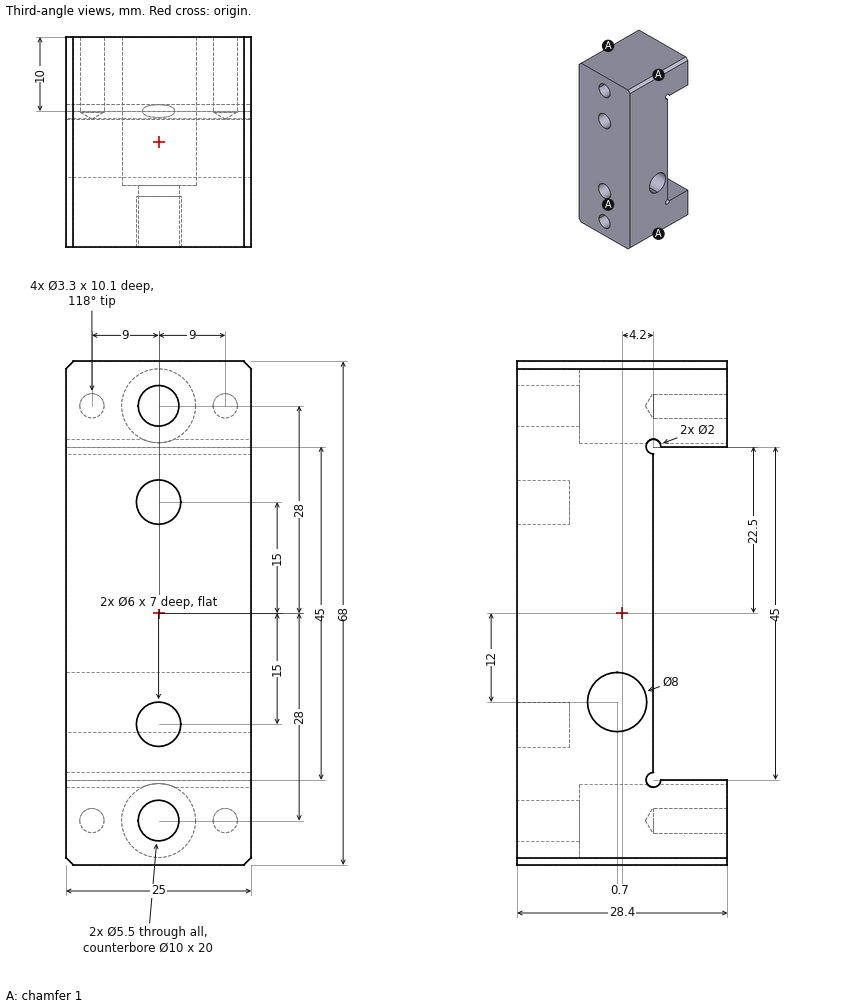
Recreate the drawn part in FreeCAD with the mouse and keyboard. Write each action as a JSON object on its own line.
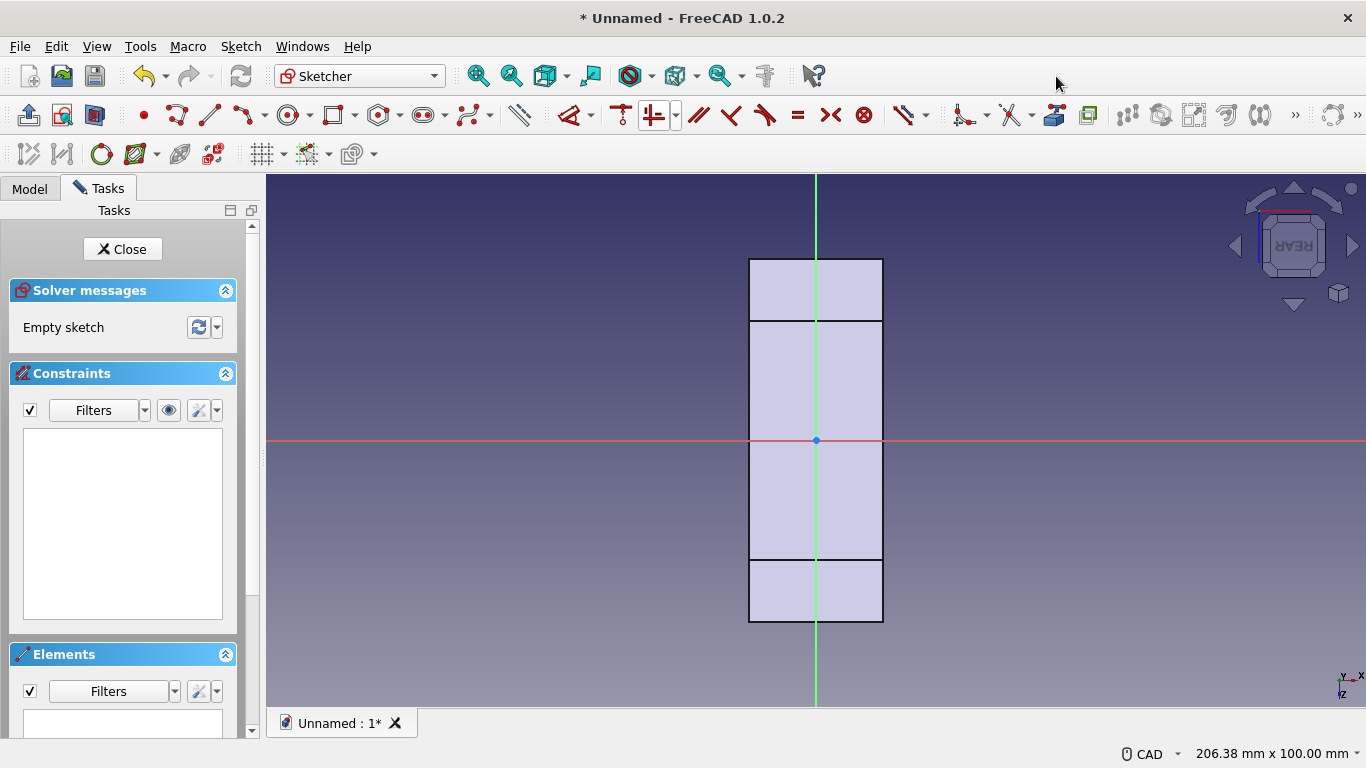
{"action": "key", "text": "g c"}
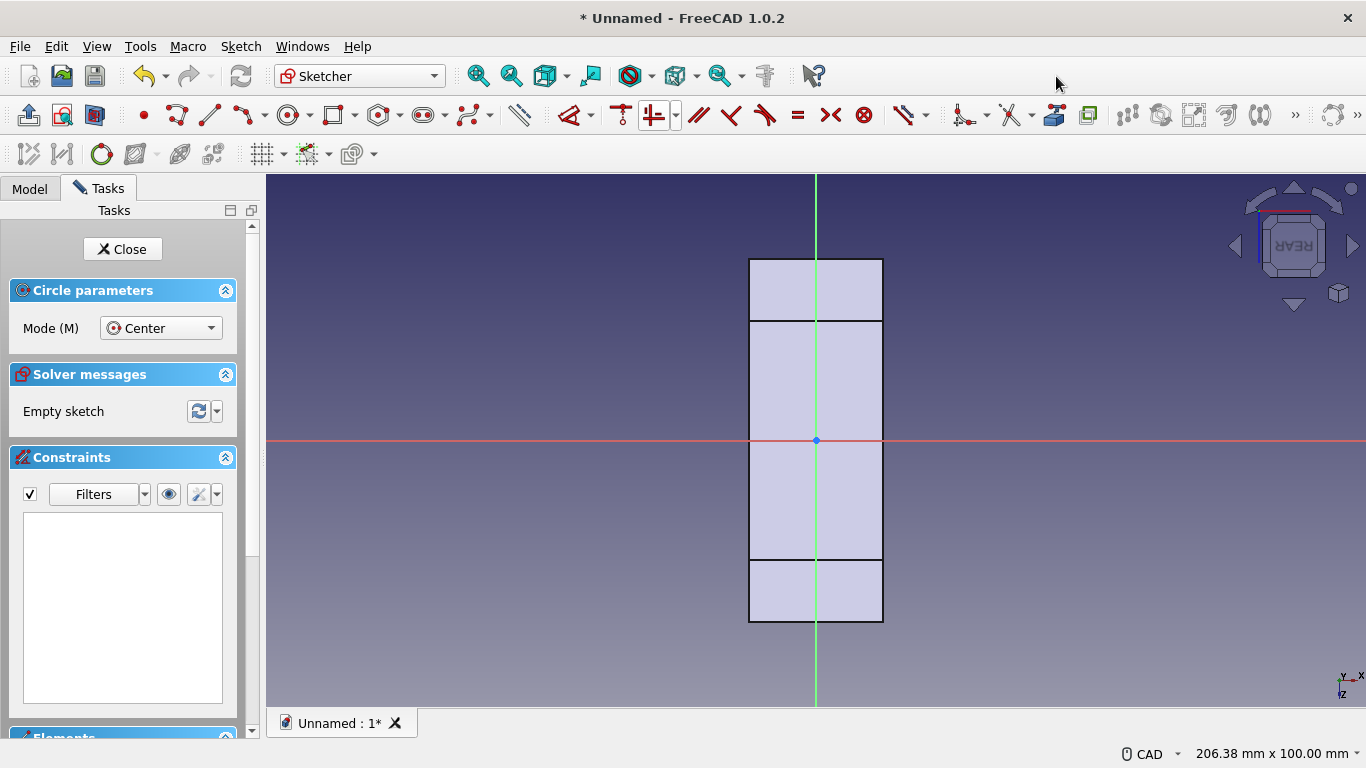
{"action": "scroll", "coordinate": [816, 291], "scroll_direction": "up", "scroll_amount": 3}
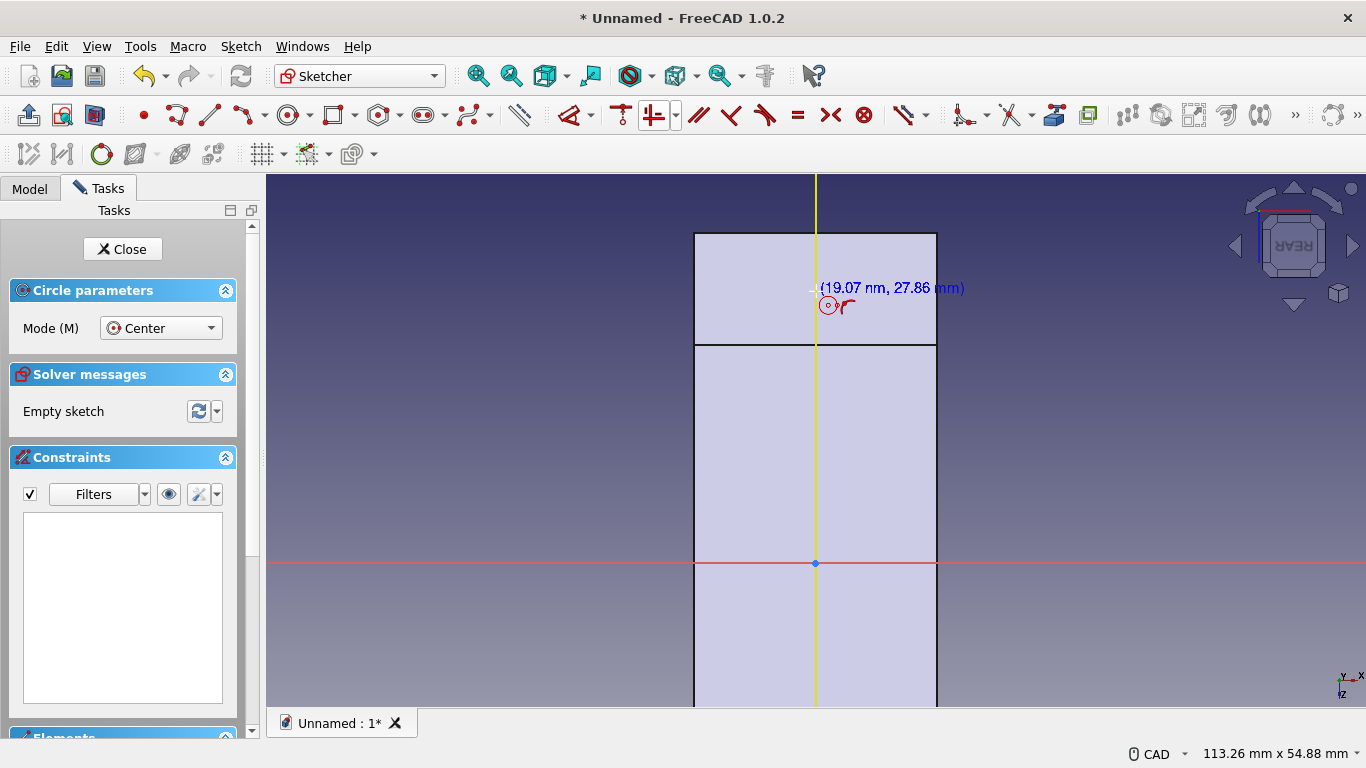
{"action": "left_click", "coordinate": [816, 291]}
{"action": "left_click", "coordinate": [834, 272]}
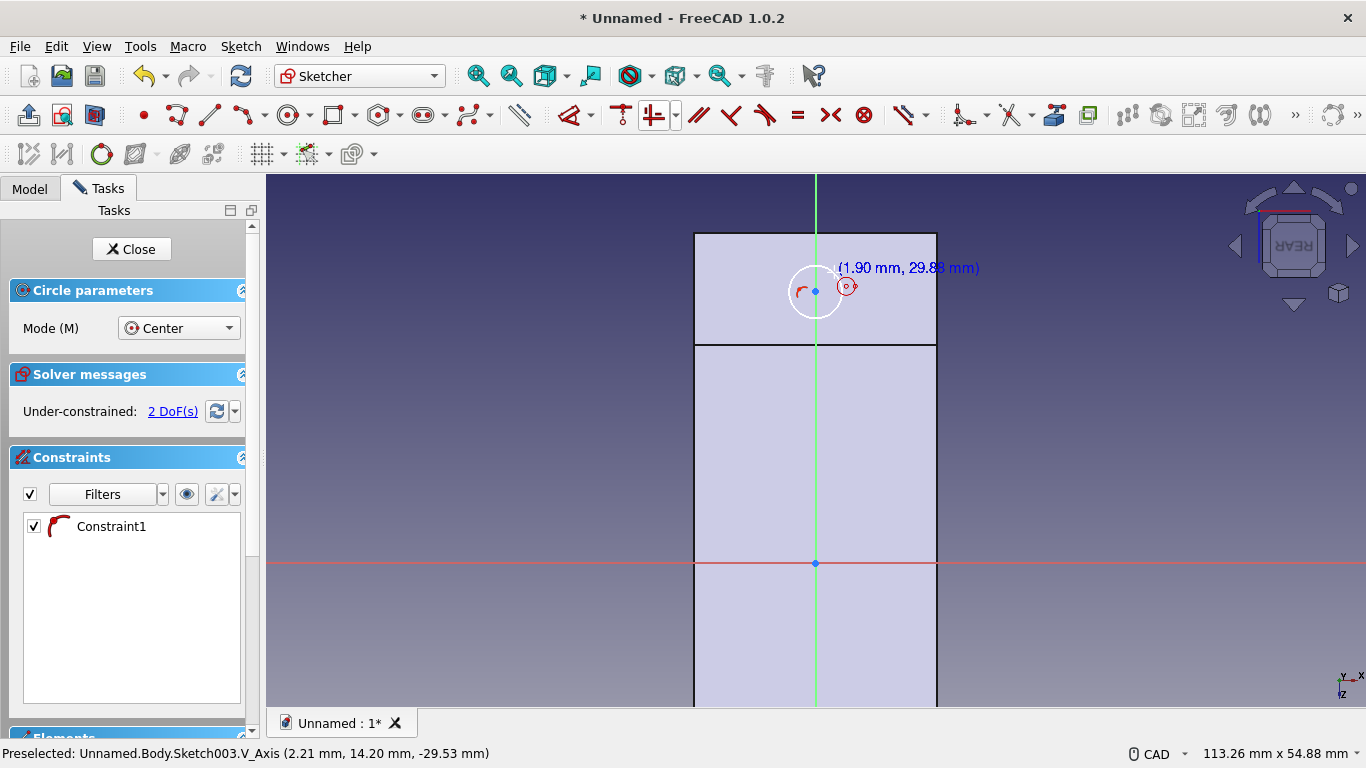
{"action": "scroll", "coordinate": [665, 291], "scroll_direction": "down", "scroll_amount": 3}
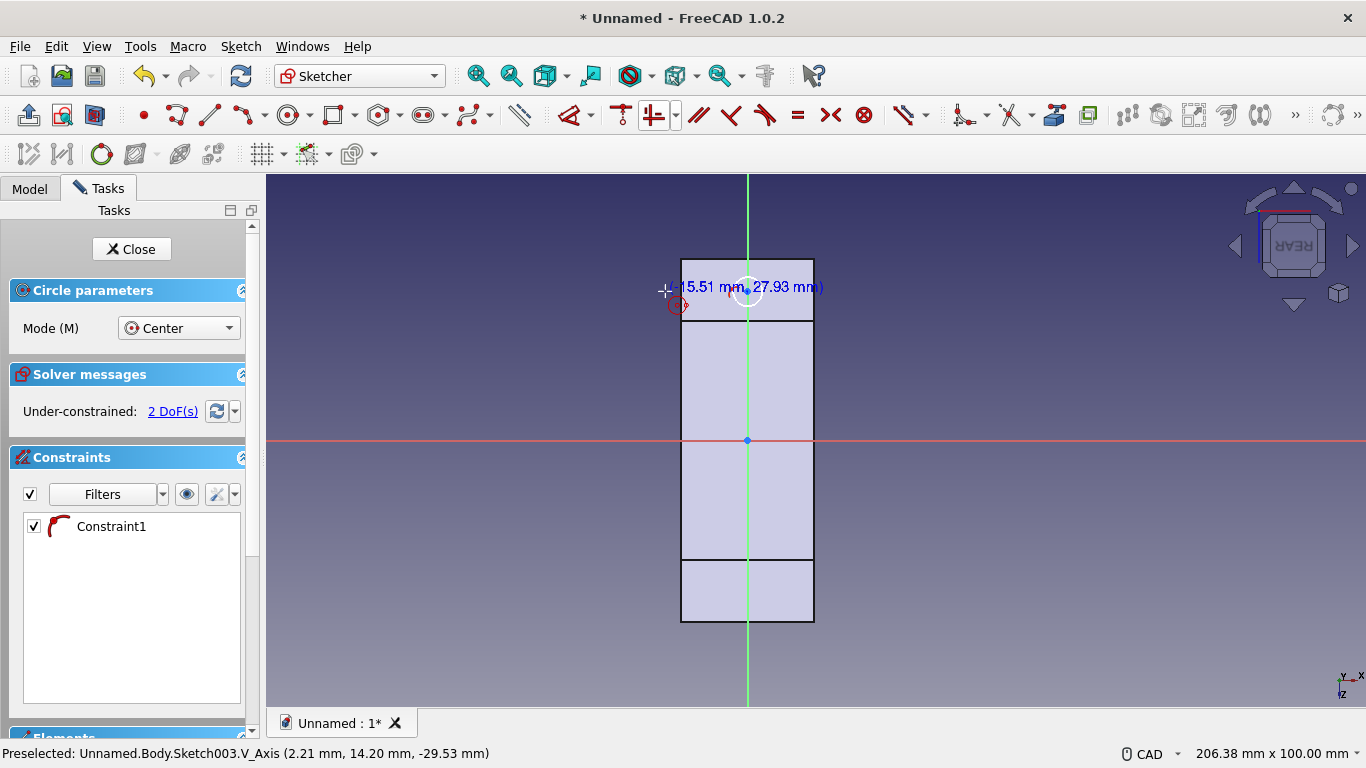
{"action": "scroll", "coordinate": [748, 590], "scroll_direction": "up", "scroll_amount": 3}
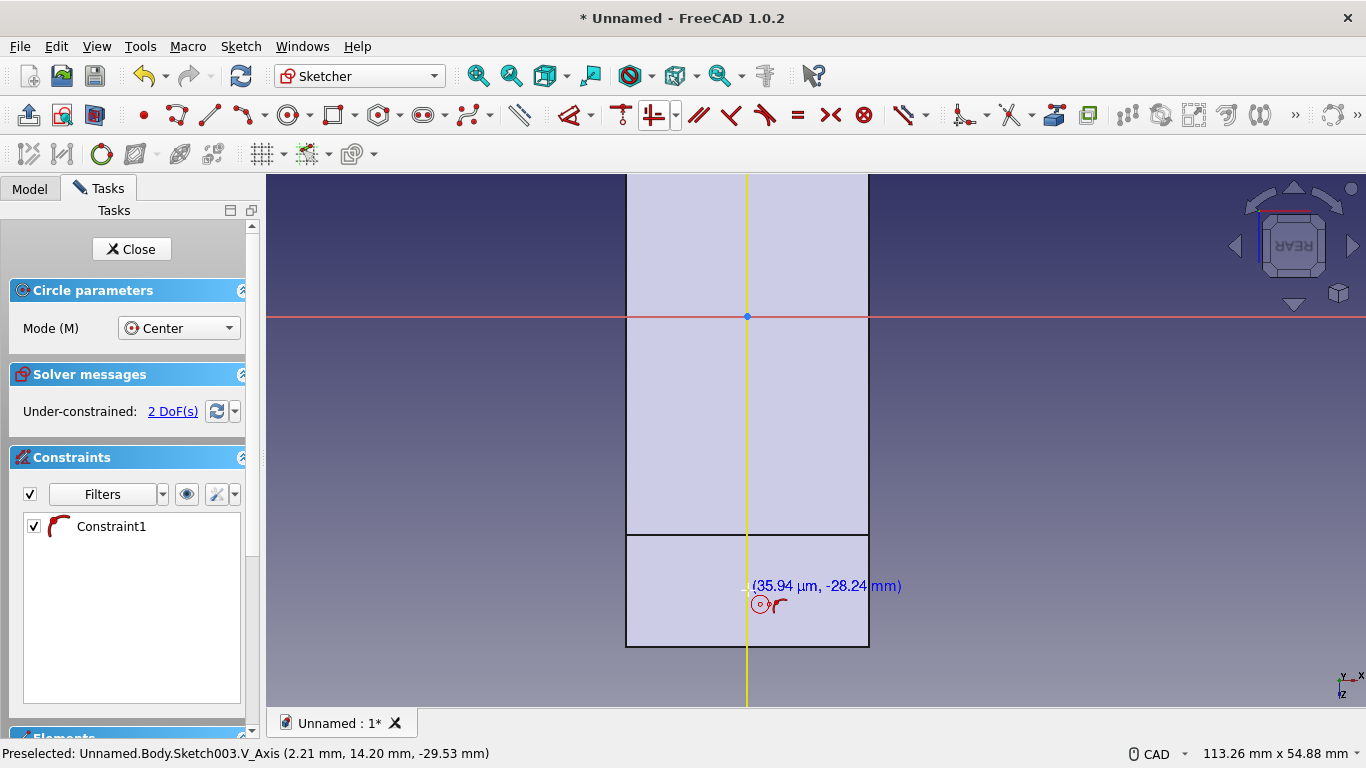
{"action": "left_click", "coordinate": [747, 589]}
{"action": "left_click", "coordinate": [766, 570]}
{"action": "key", "text": "Escape"}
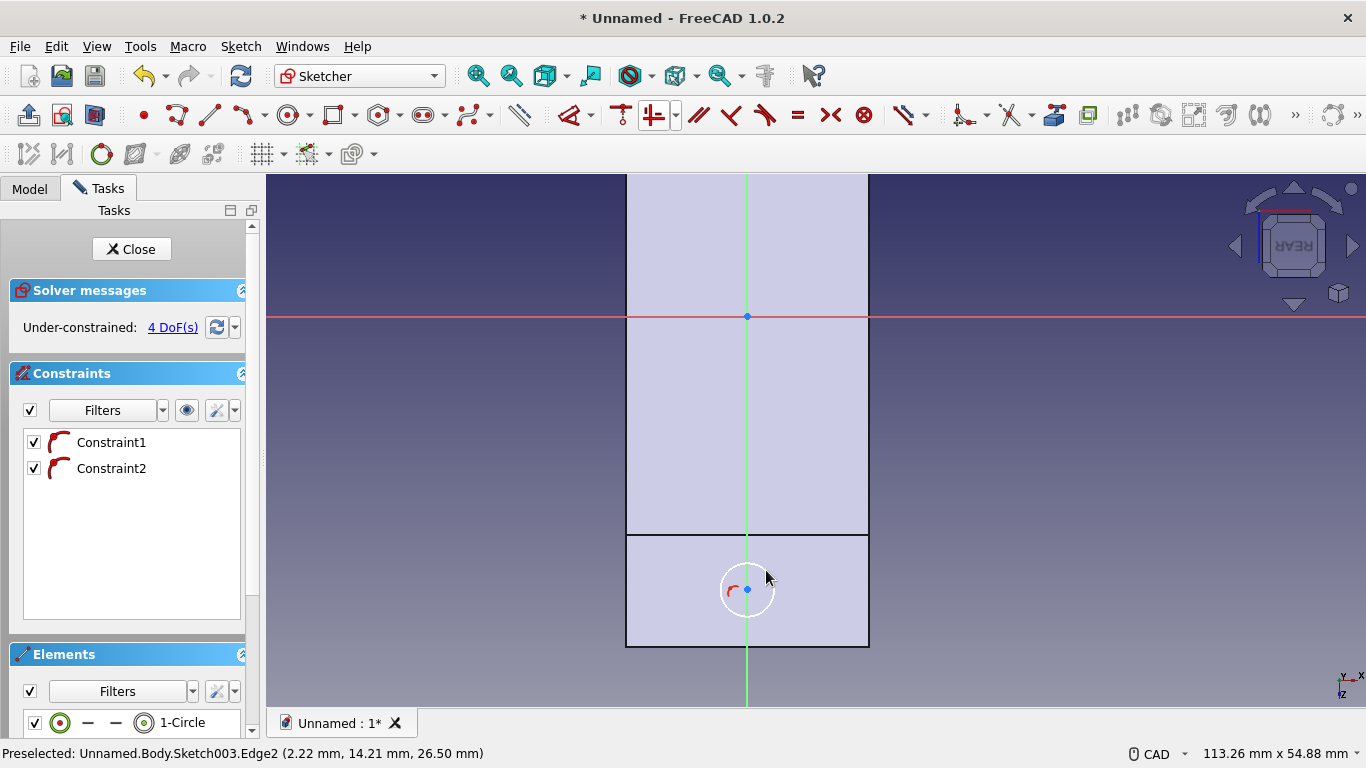
{"action": "scroll", "coordinate": [748, 591], "scroll_direction": "down", "scroll_amount": 3}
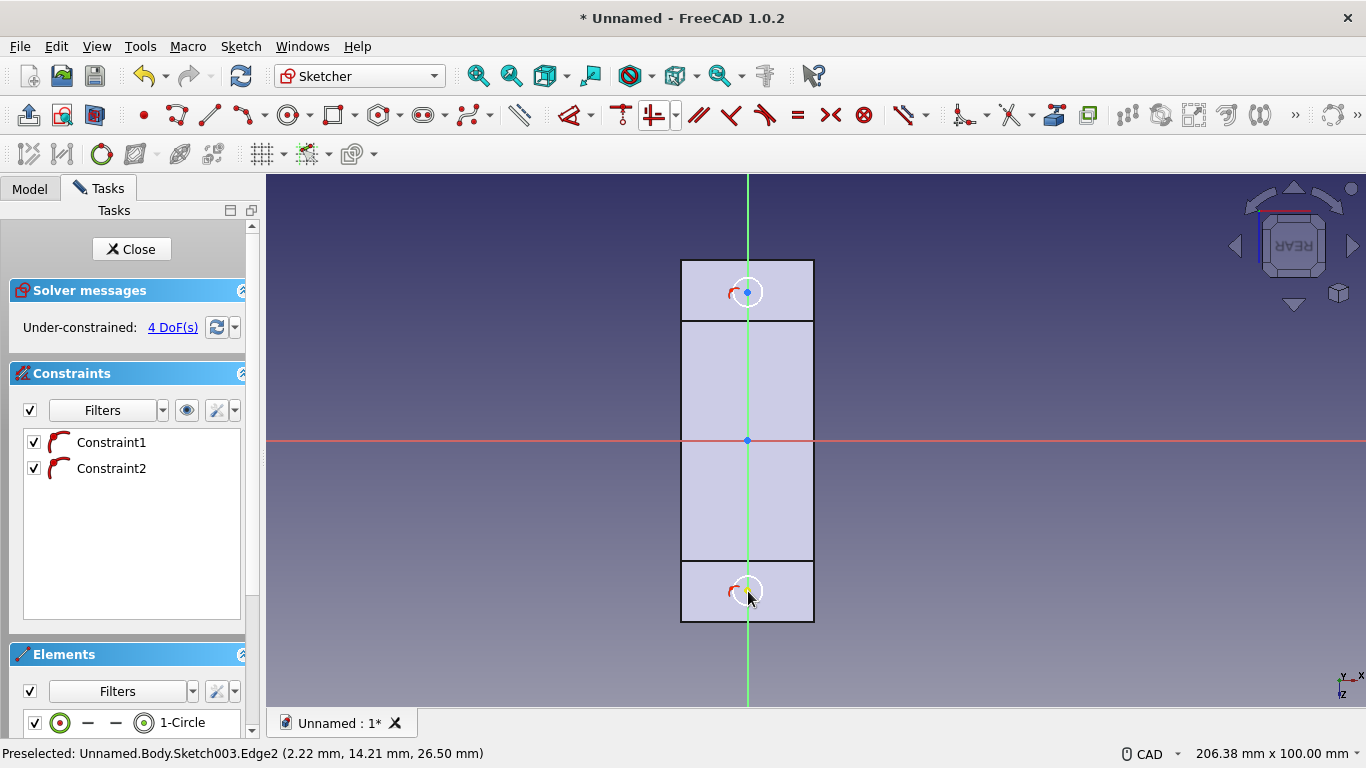
{"action": "scroll", "coordinate": [758, 282], "scroll_direction": "up", "scroll_amount": 2}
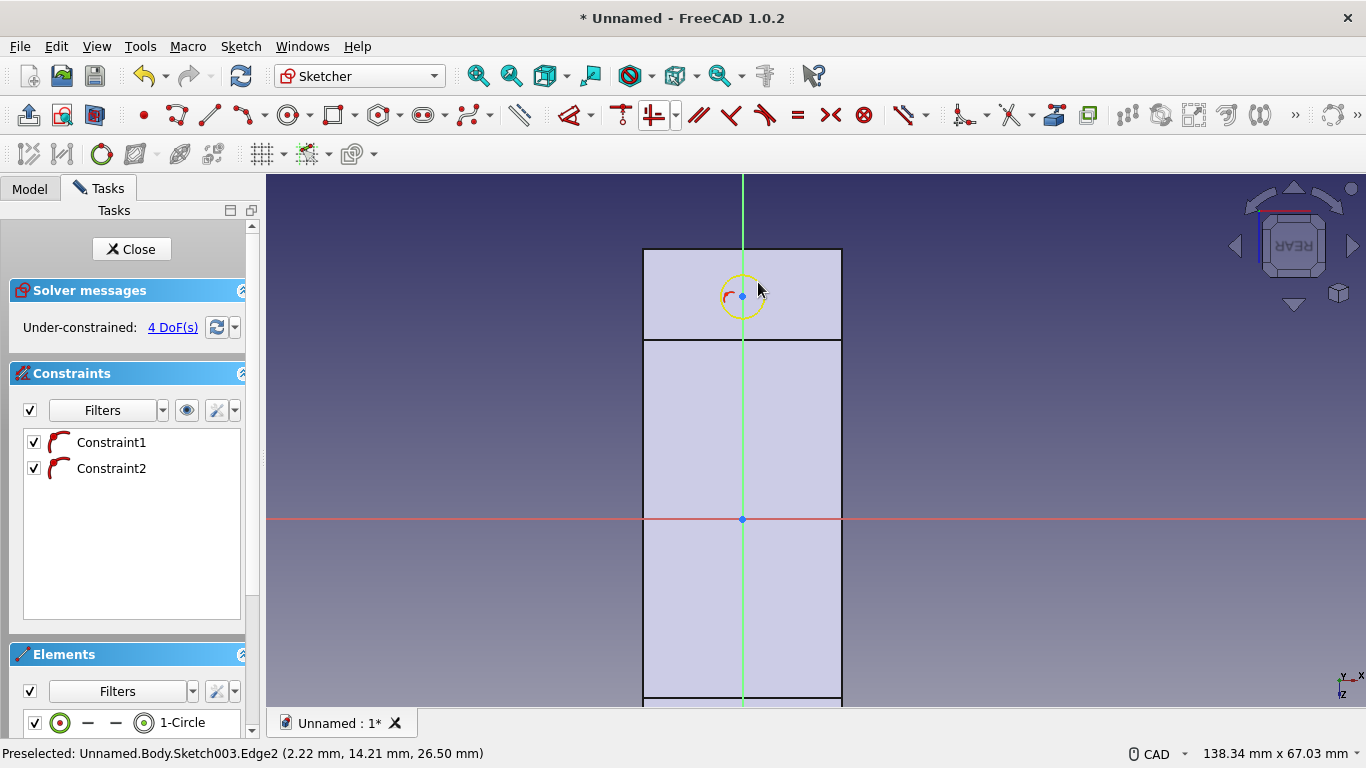
{"action": "left_click", "coordinate": [758, 282]}